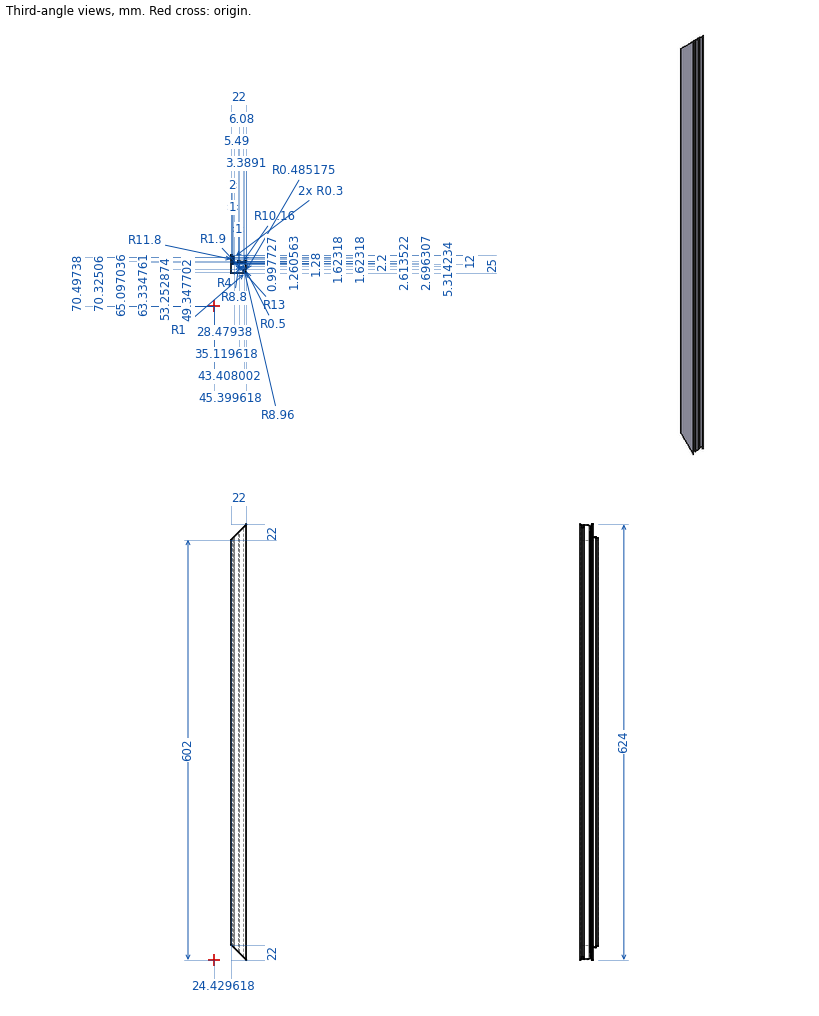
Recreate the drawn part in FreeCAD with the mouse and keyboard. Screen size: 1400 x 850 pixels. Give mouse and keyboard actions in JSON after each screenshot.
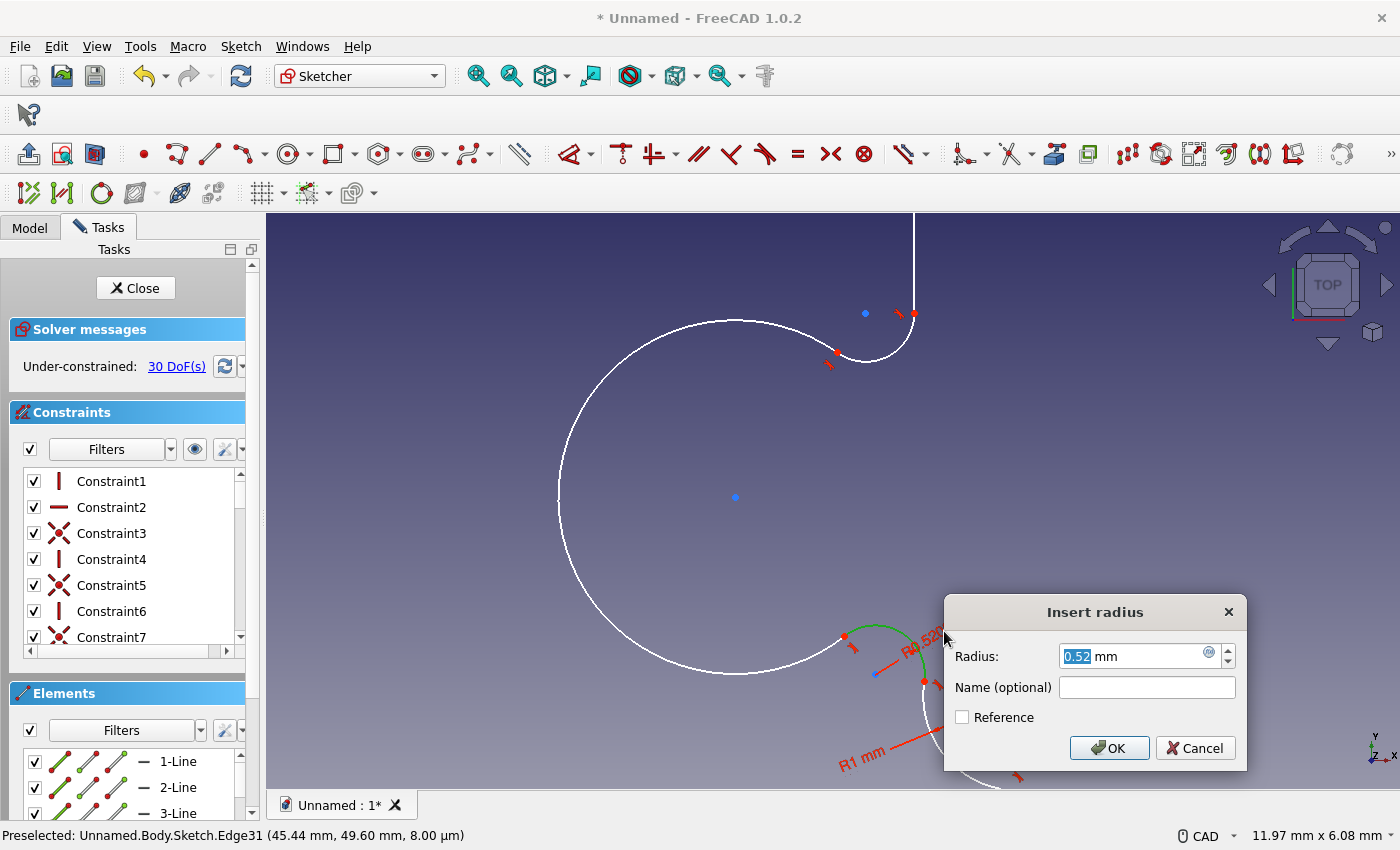
{"action": "type", "text": "0.485175"}
{"action": "key", "text": "Return"}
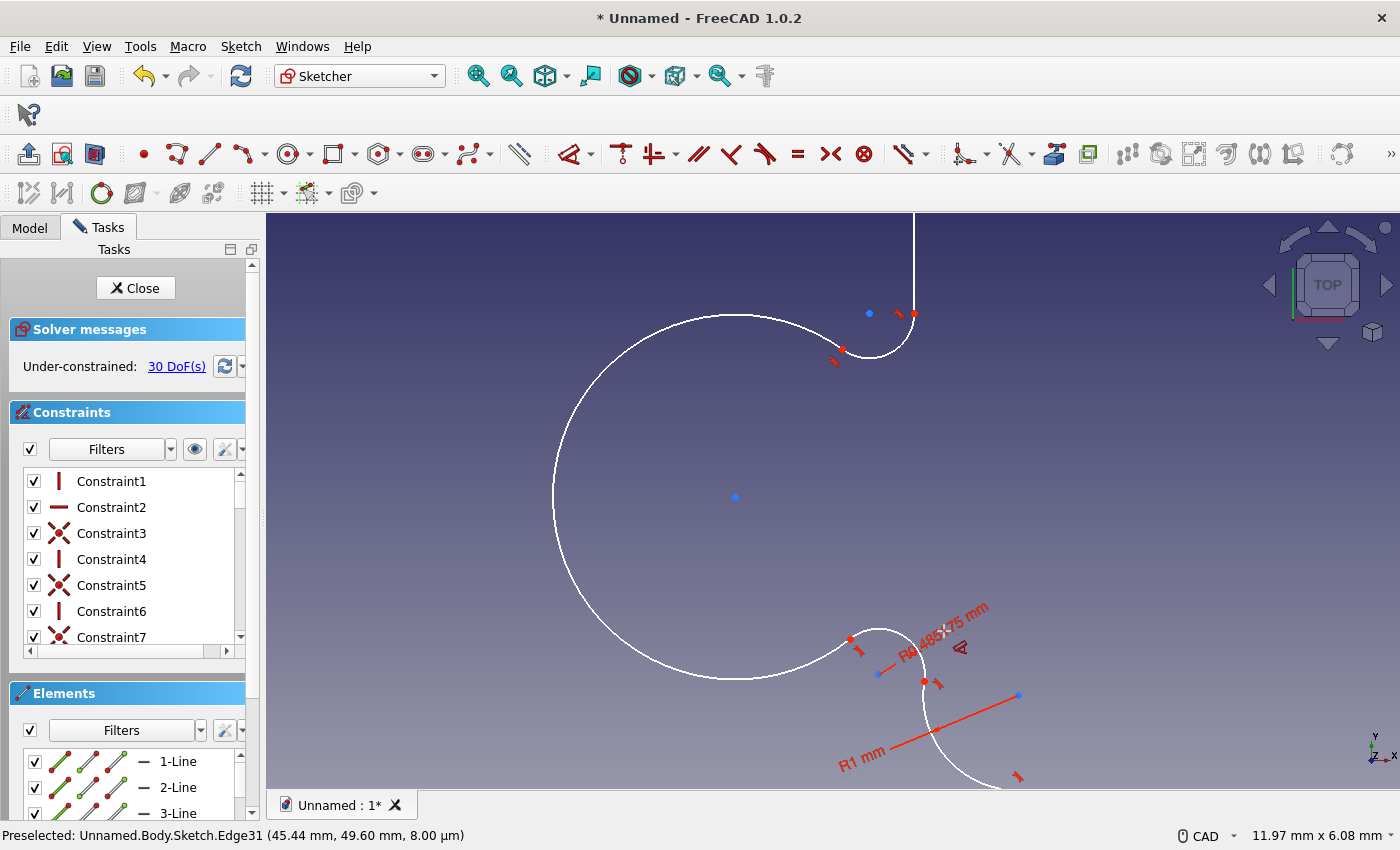
{"action": "scroll", "coordinate": [922, 679], "scroll_direction": "down", "scroll_amount": 9}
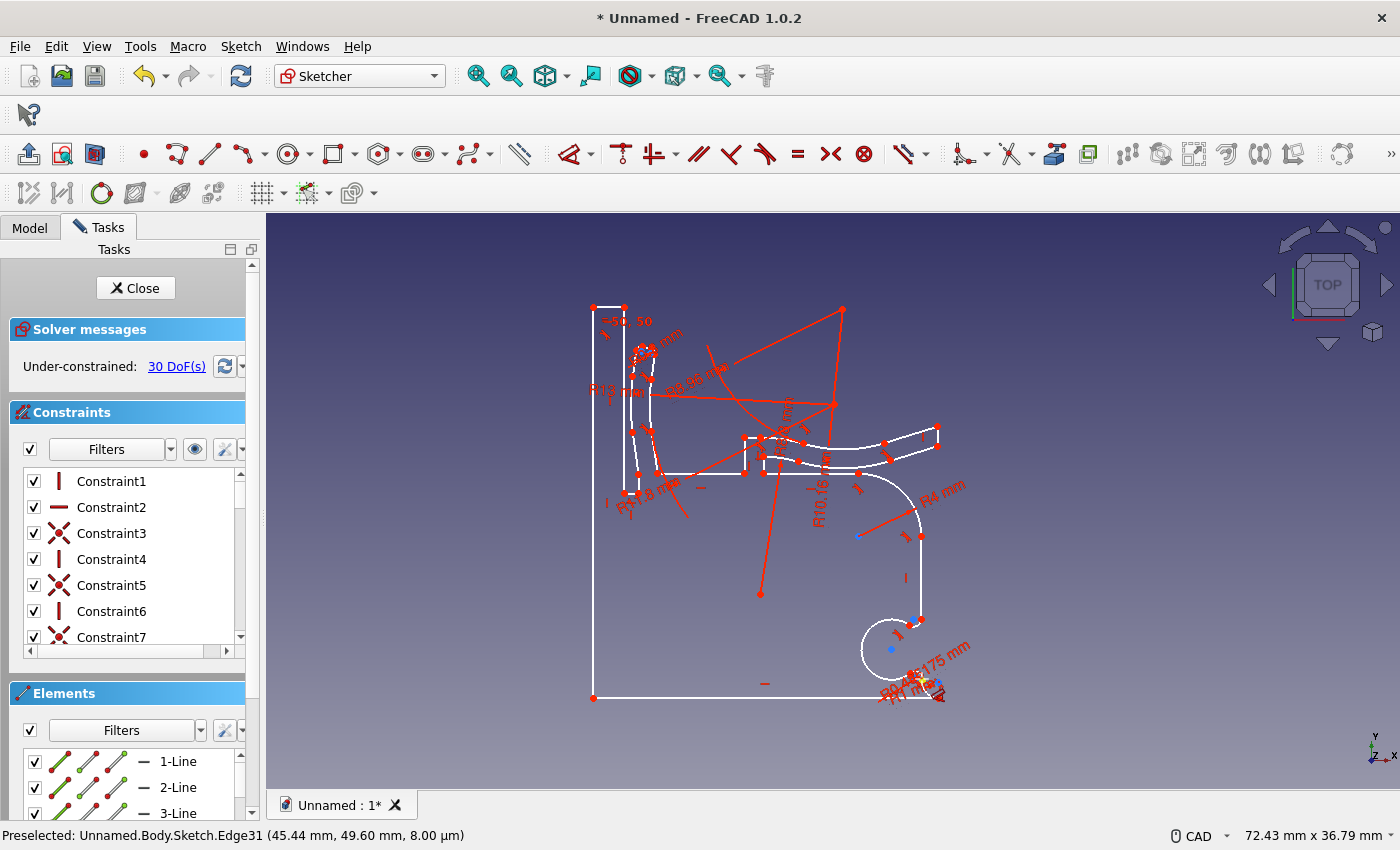
{"action": "scroll", "coordinate": [872, 627], "scroll_direction": "up", "scroll_amount": 2}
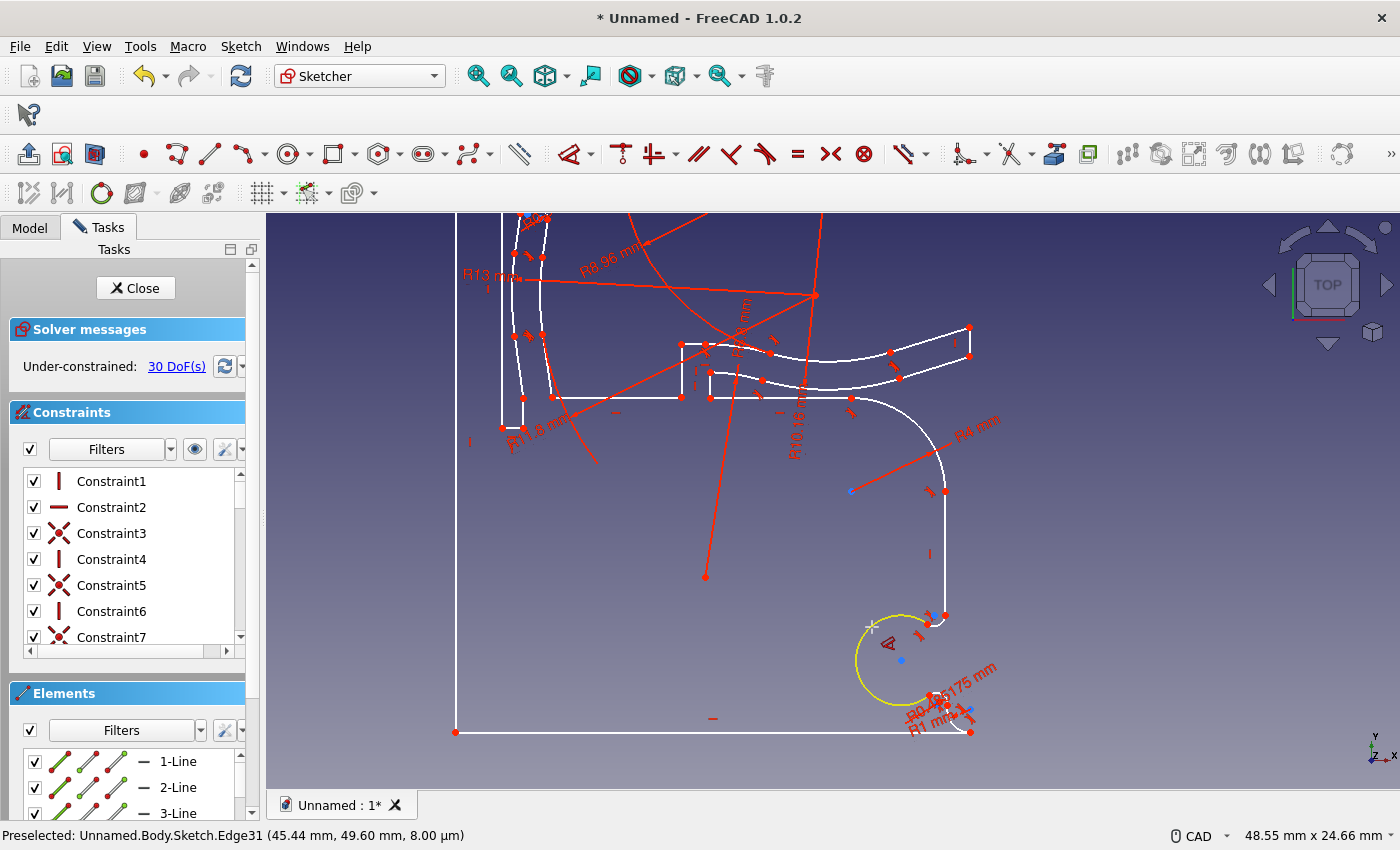
{"action": "left_click", "coordinate": [872, 626]}
{"action": "left_click", "coordinate": [851, 602]}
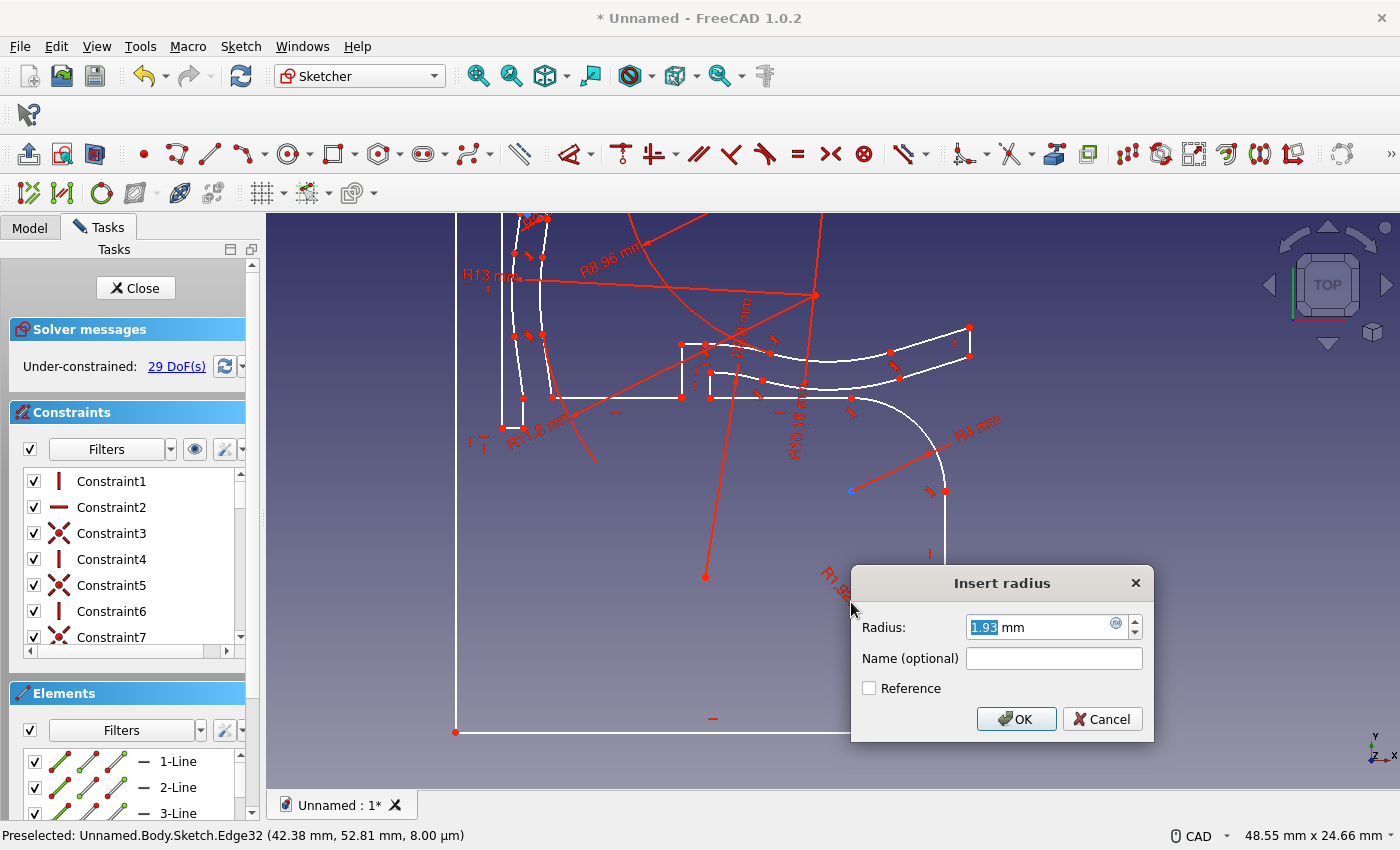
{"action": "type", "text": "1.9"}
{"action": "key", "text": "Return"}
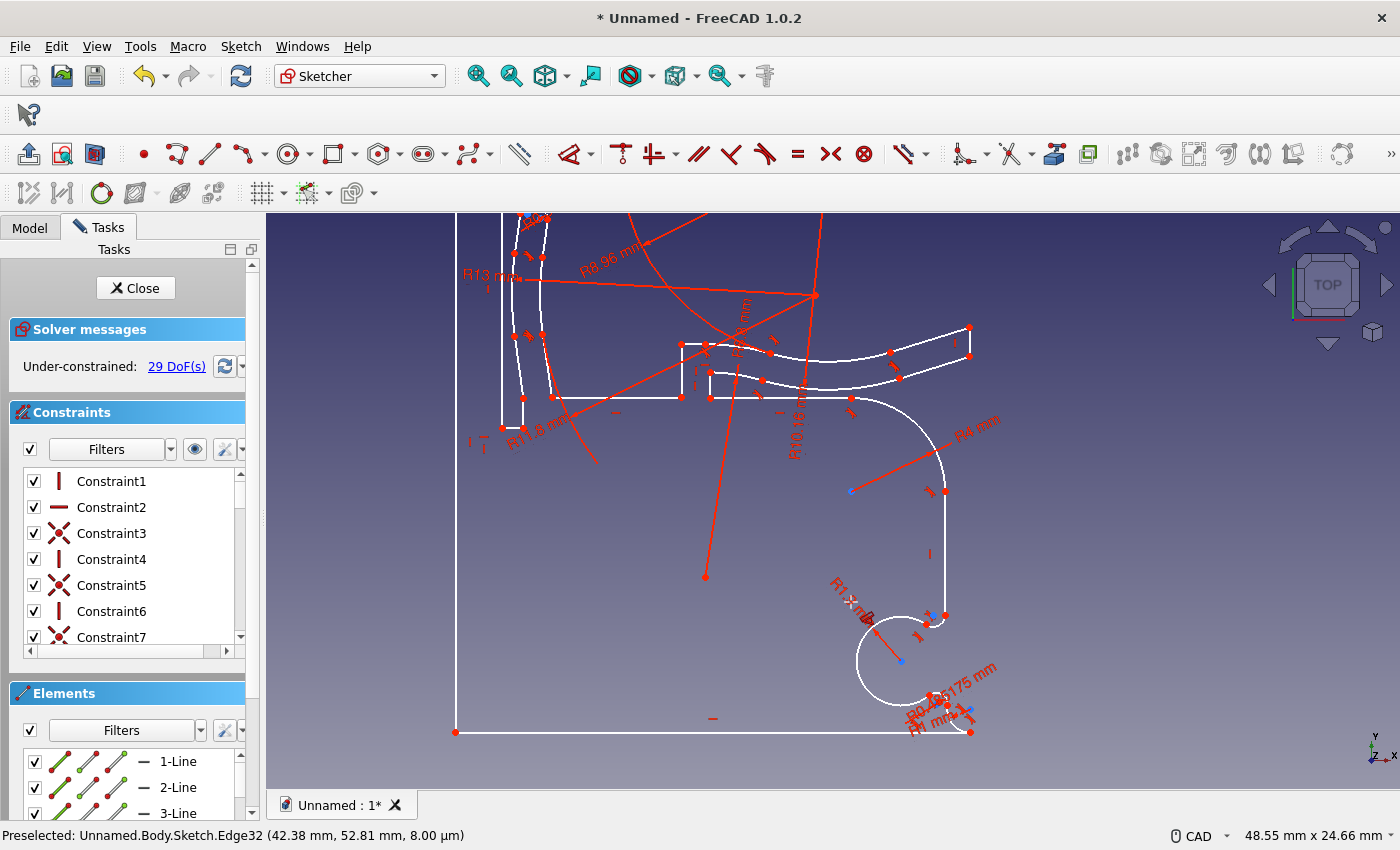
{"action": "scroll", "coordinate": [939, 626], "scroll_direction": "up", "scroll_amount": 7}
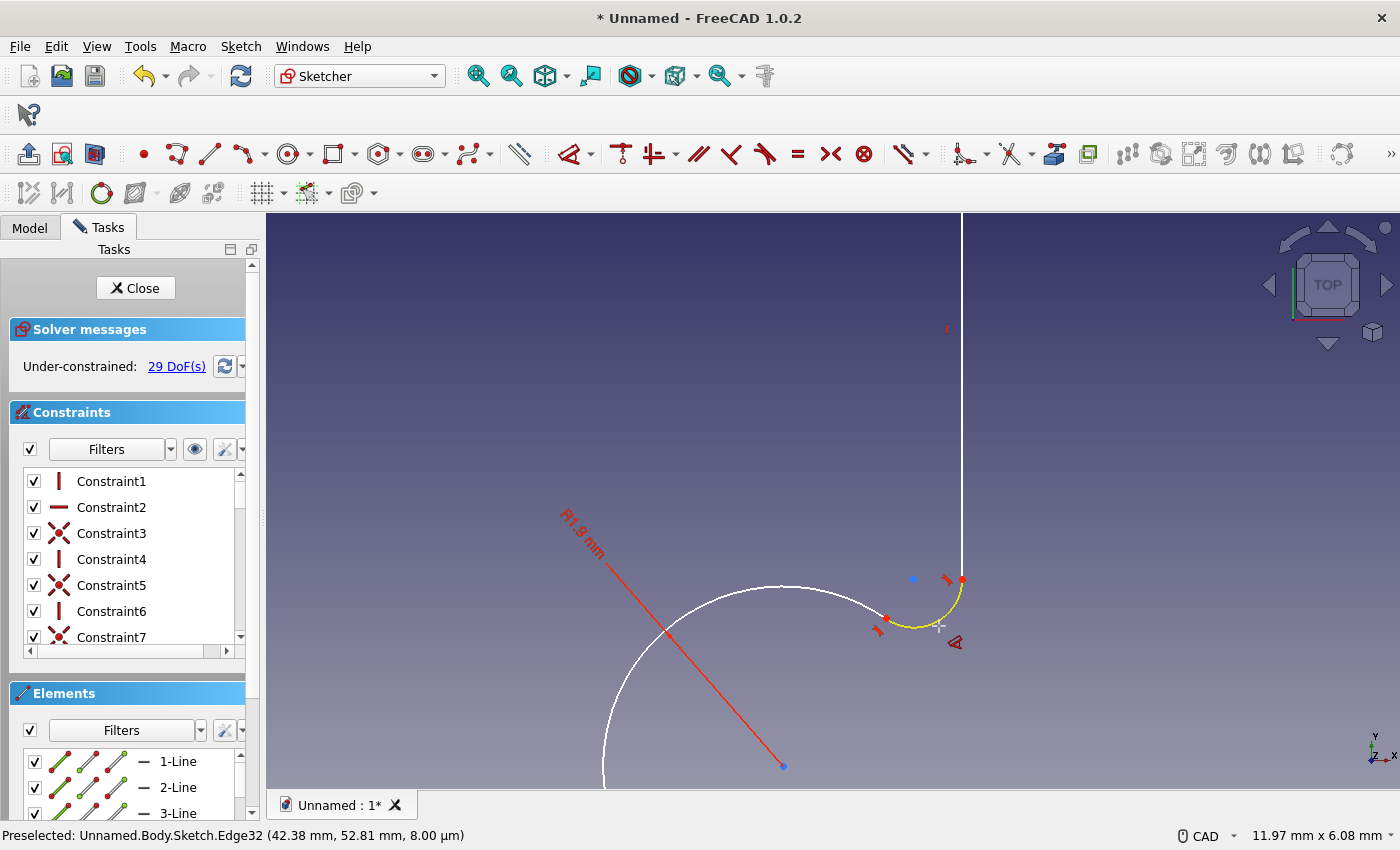
{"action": "left_click", "coordinate": [936, 622]}
{"action": "left_click", "coordinate": [951, 650]}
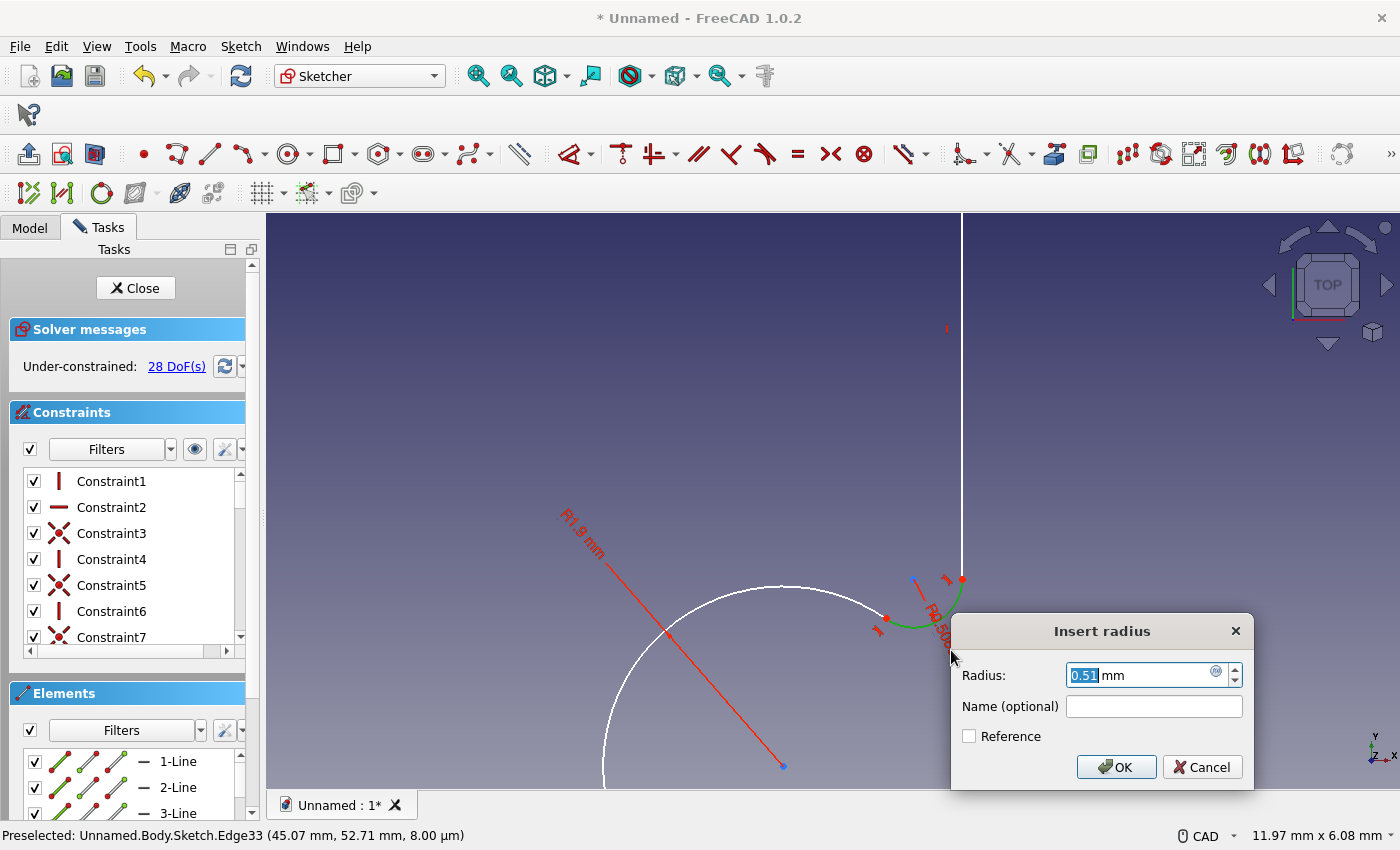
{"action": "type", "text": "0.5"}
{"action": "key", "text": "Return"}